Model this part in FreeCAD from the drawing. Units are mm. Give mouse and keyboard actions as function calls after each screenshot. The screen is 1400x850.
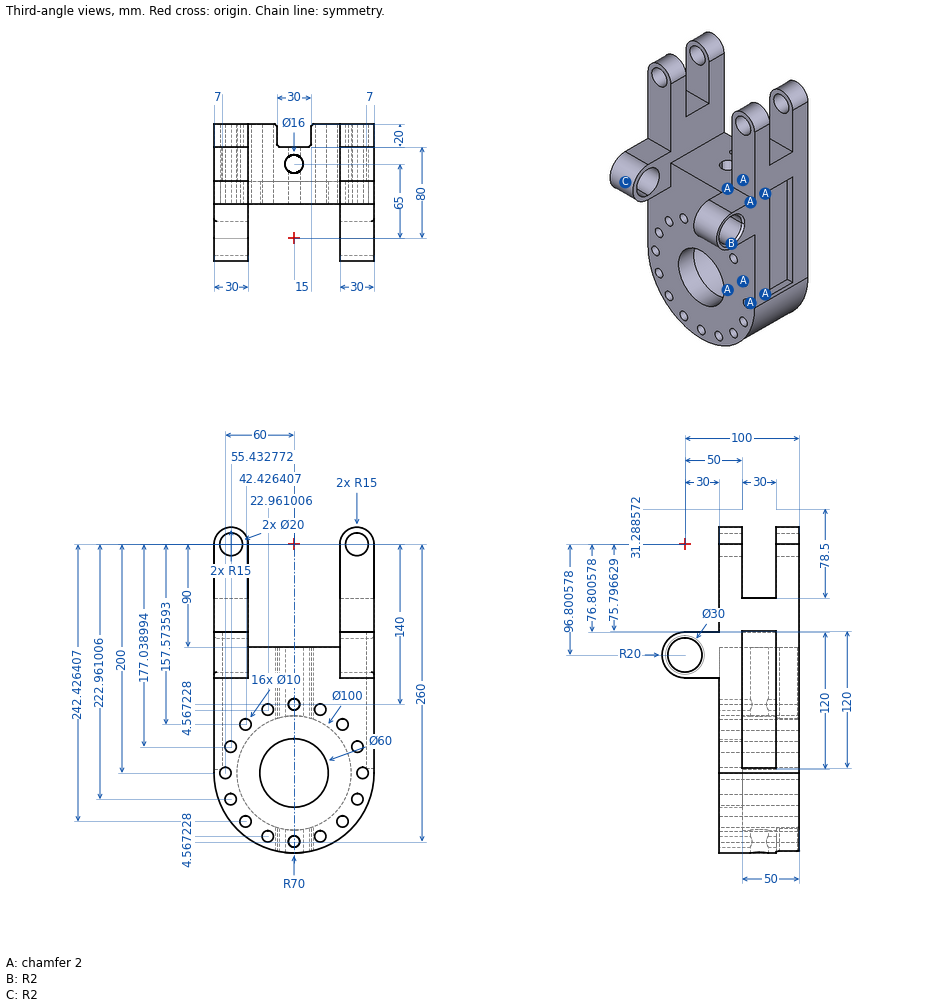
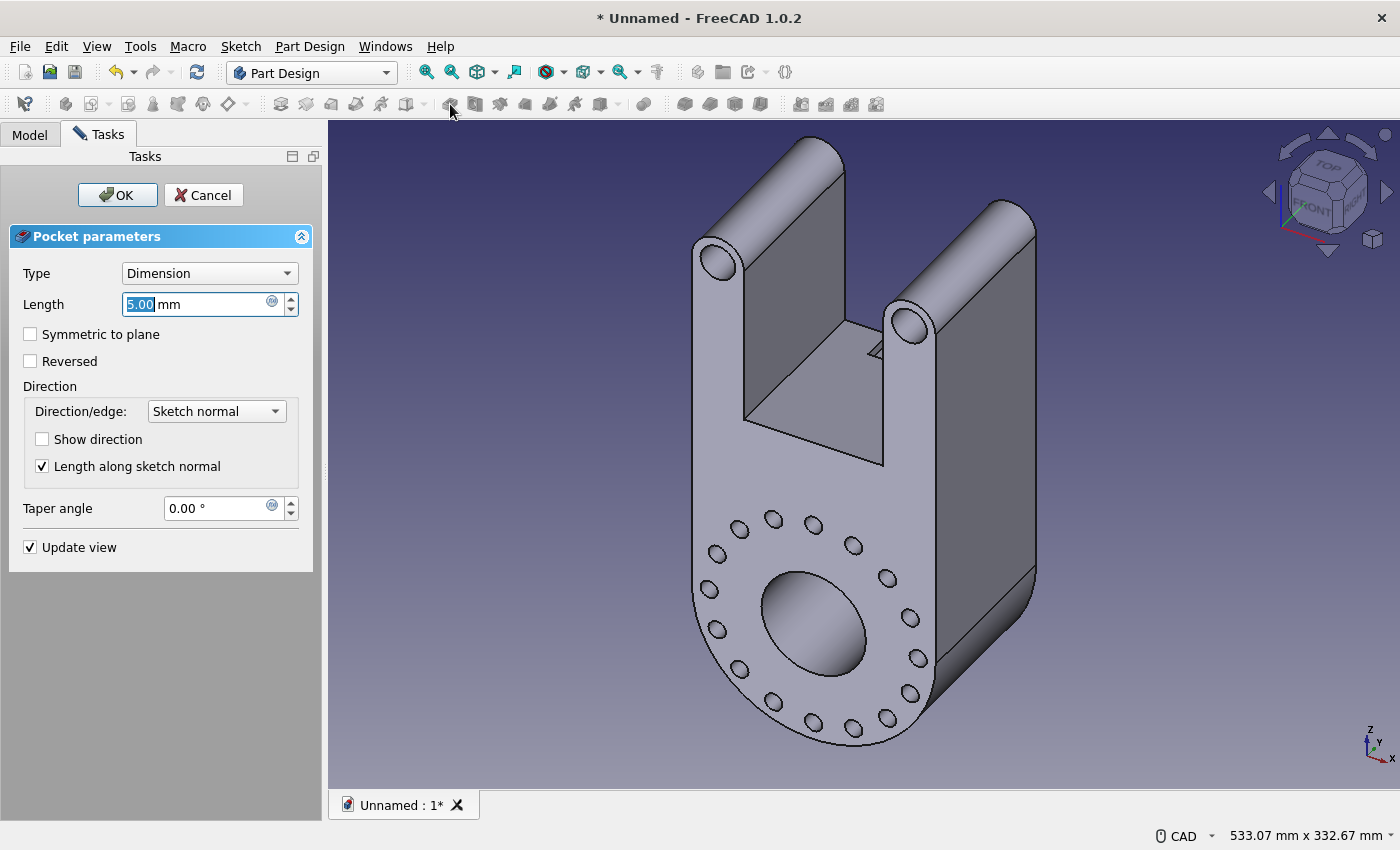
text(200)
key(Tab)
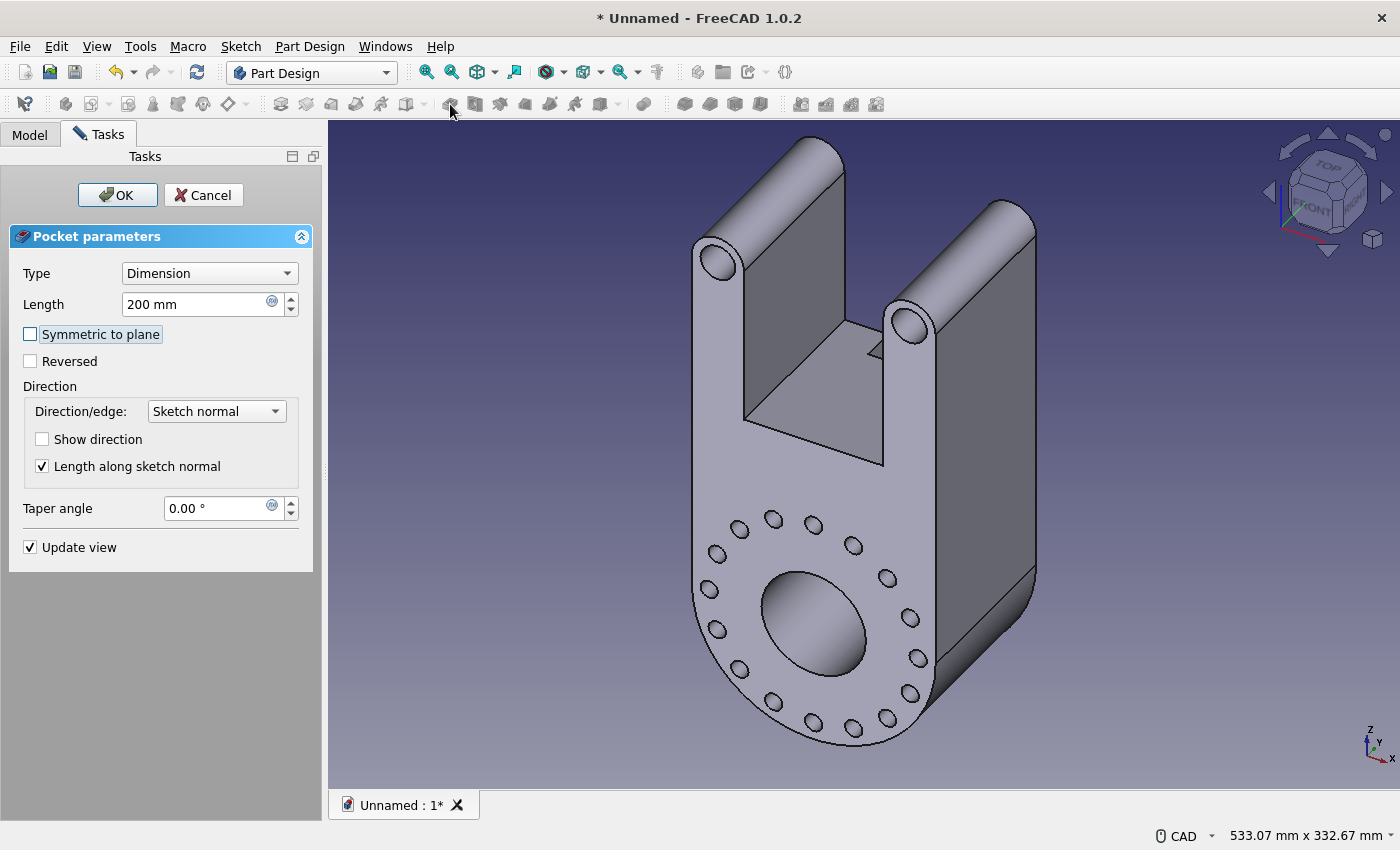
click(118, 195)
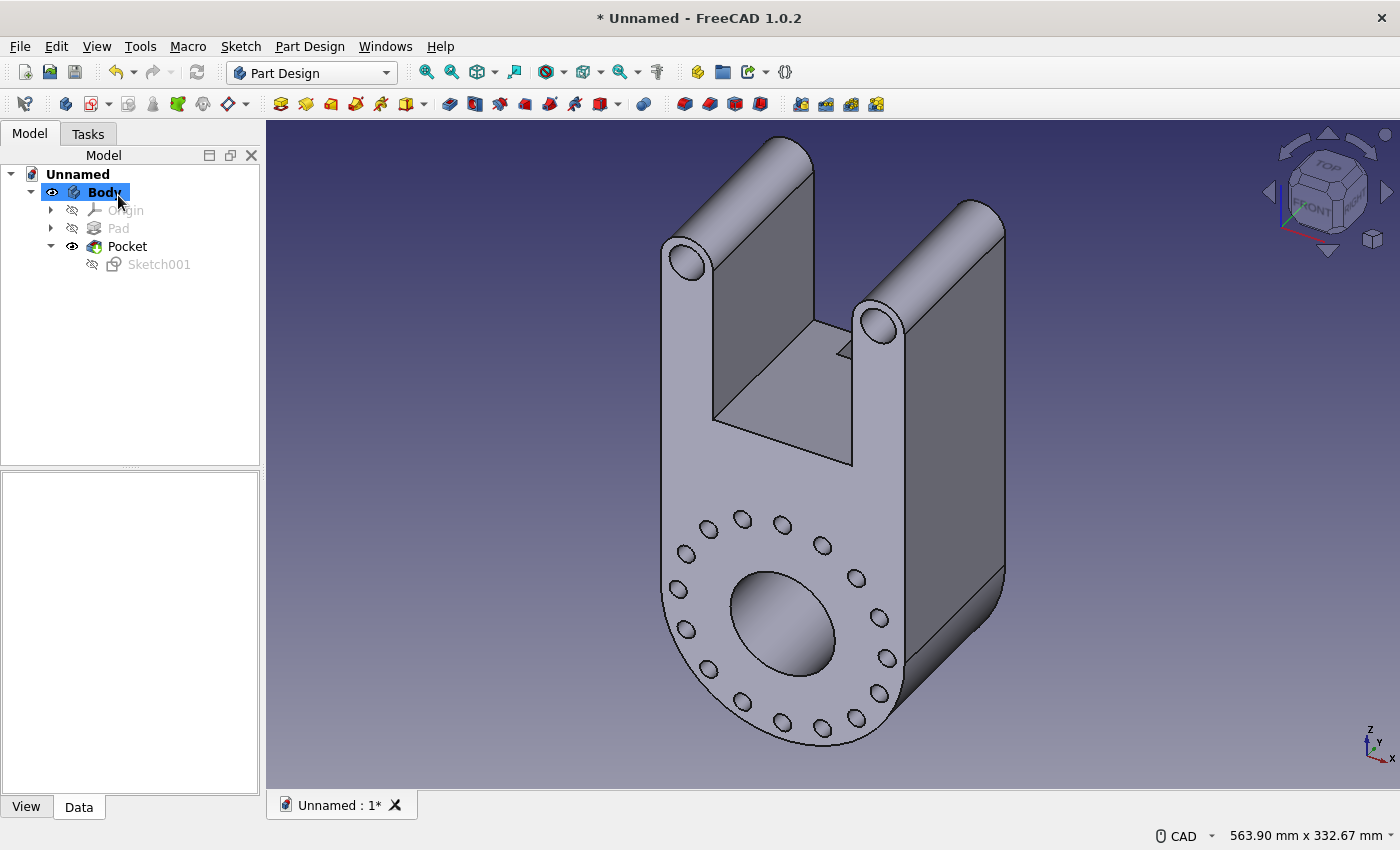
key(0)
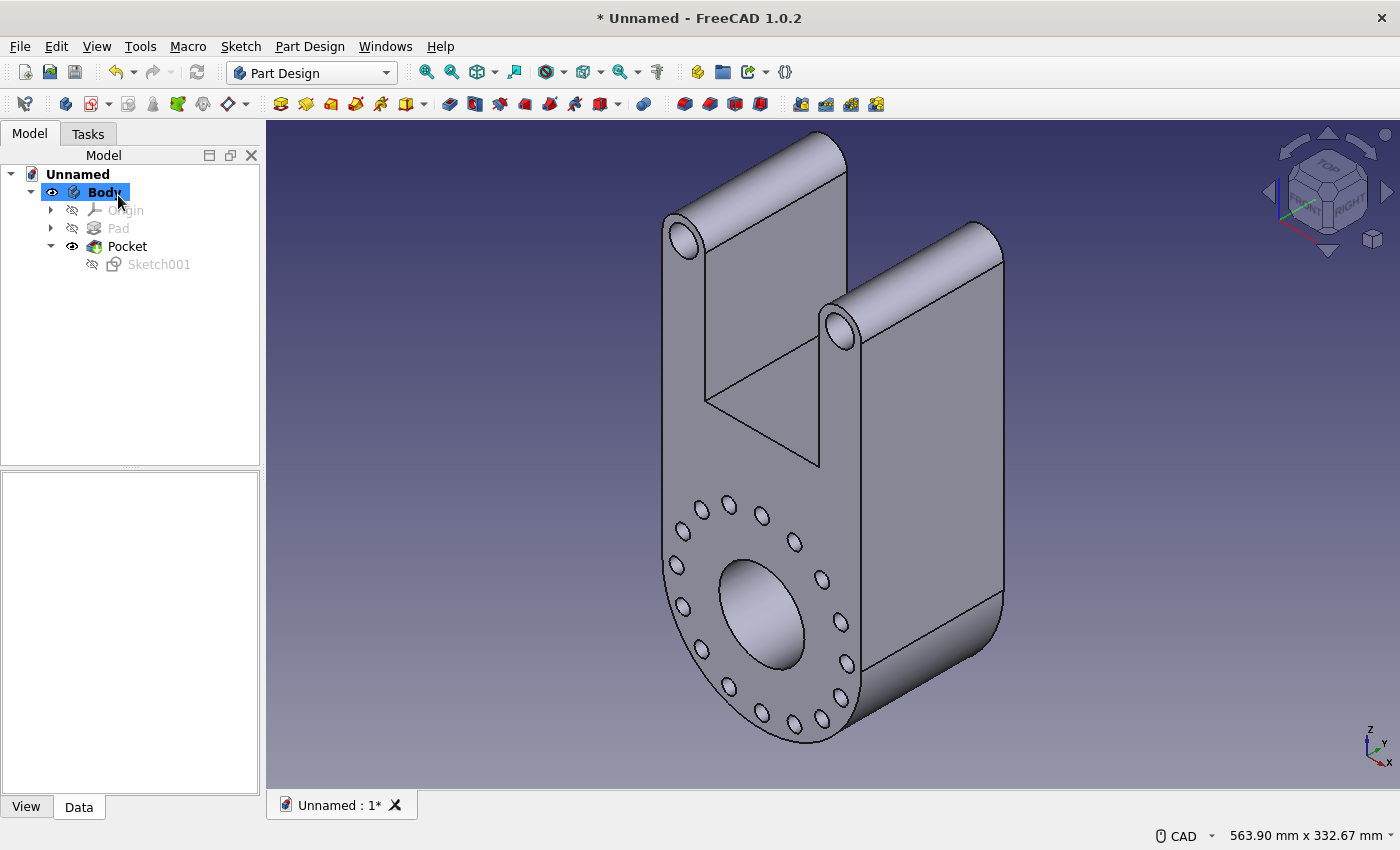
key(2)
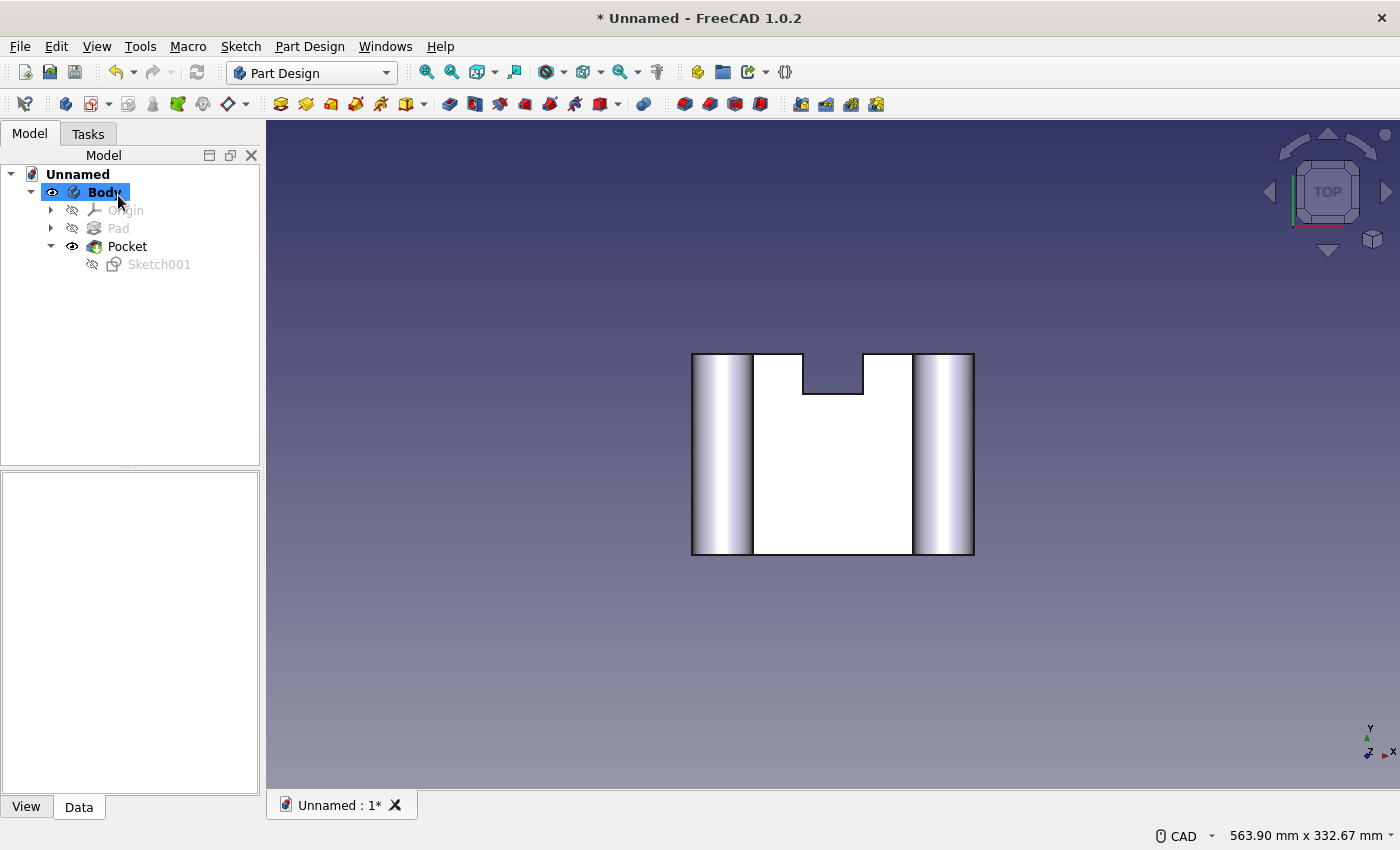
key(v)
key(f)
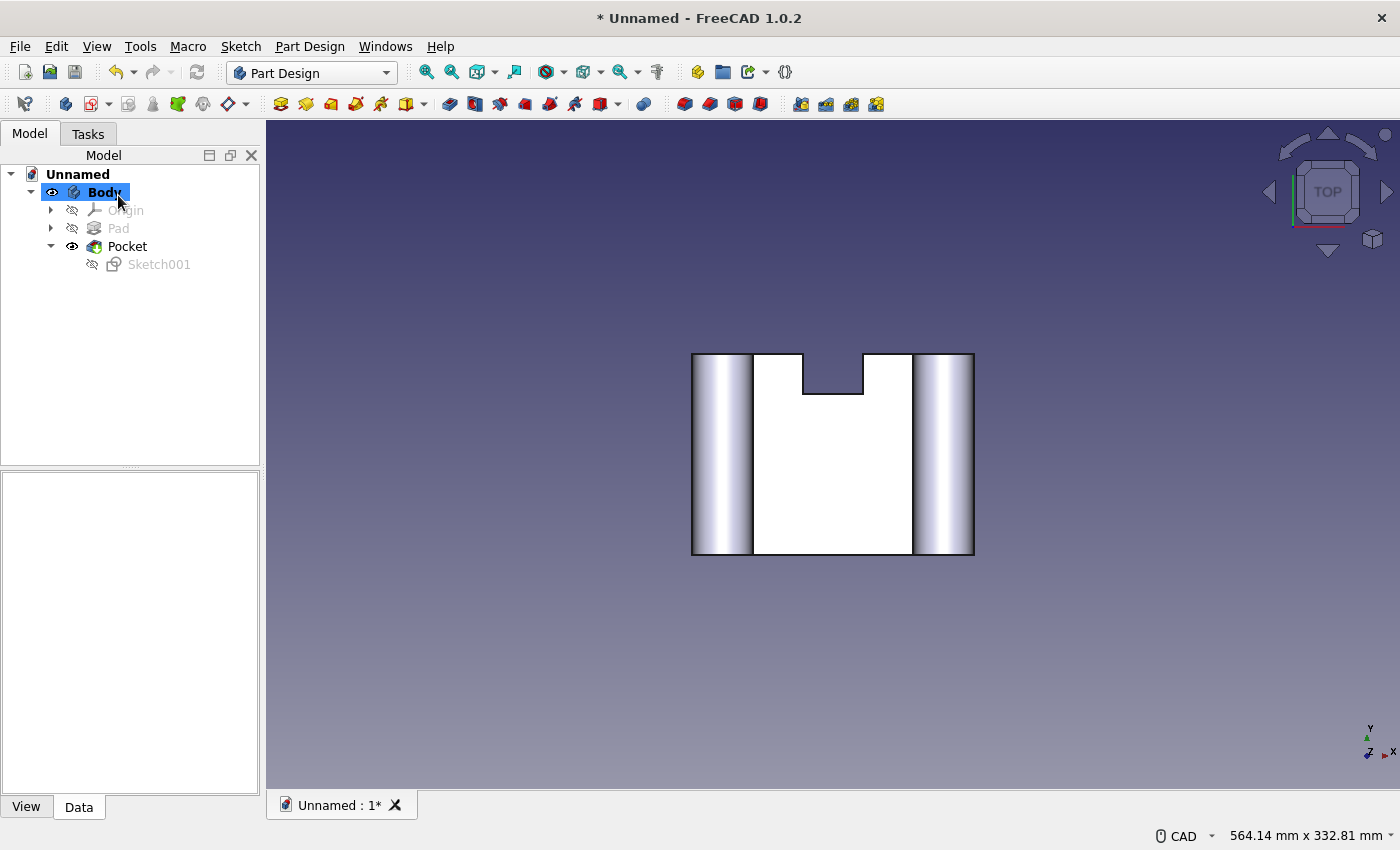
key(1)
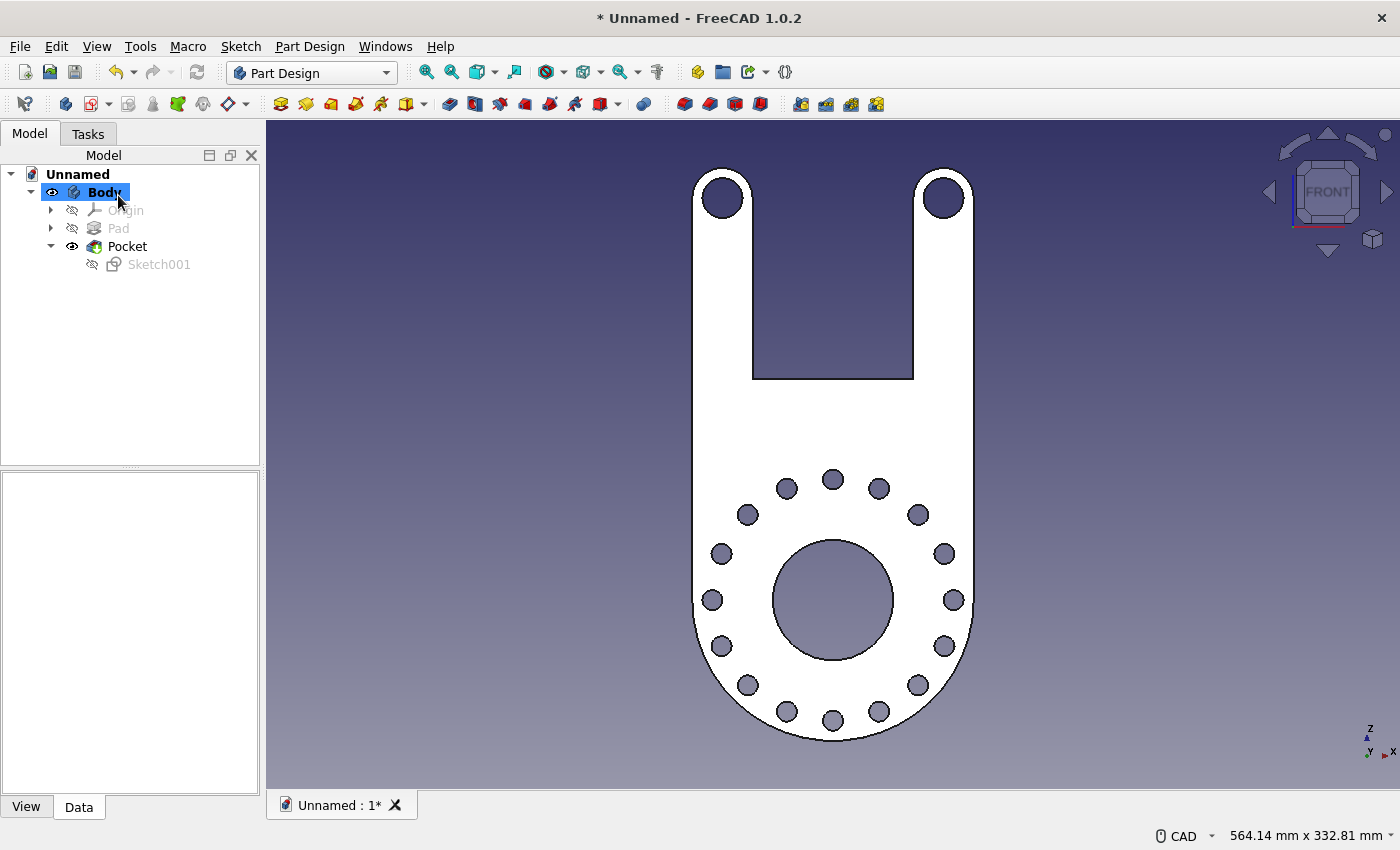
key(3)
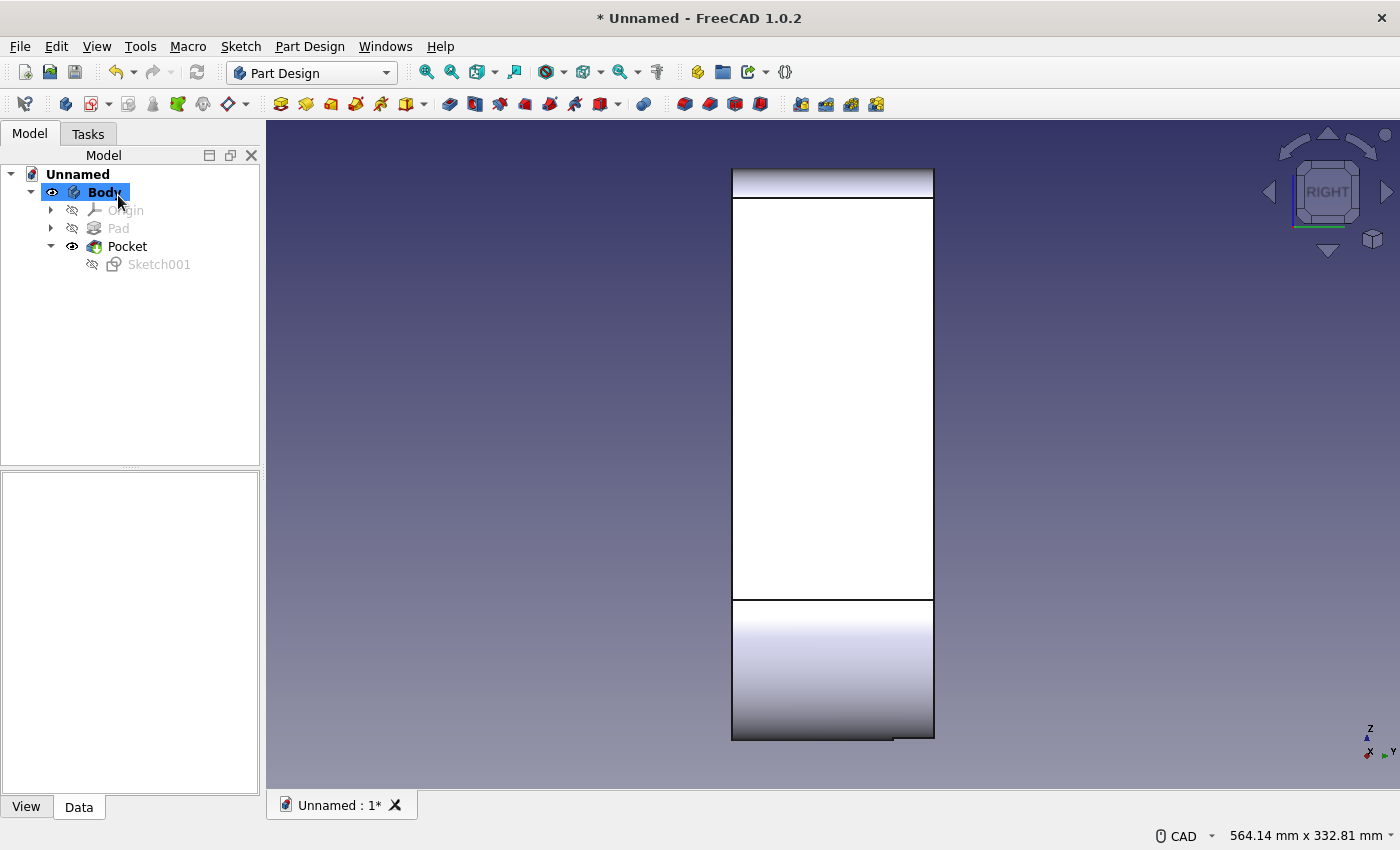
key(5)